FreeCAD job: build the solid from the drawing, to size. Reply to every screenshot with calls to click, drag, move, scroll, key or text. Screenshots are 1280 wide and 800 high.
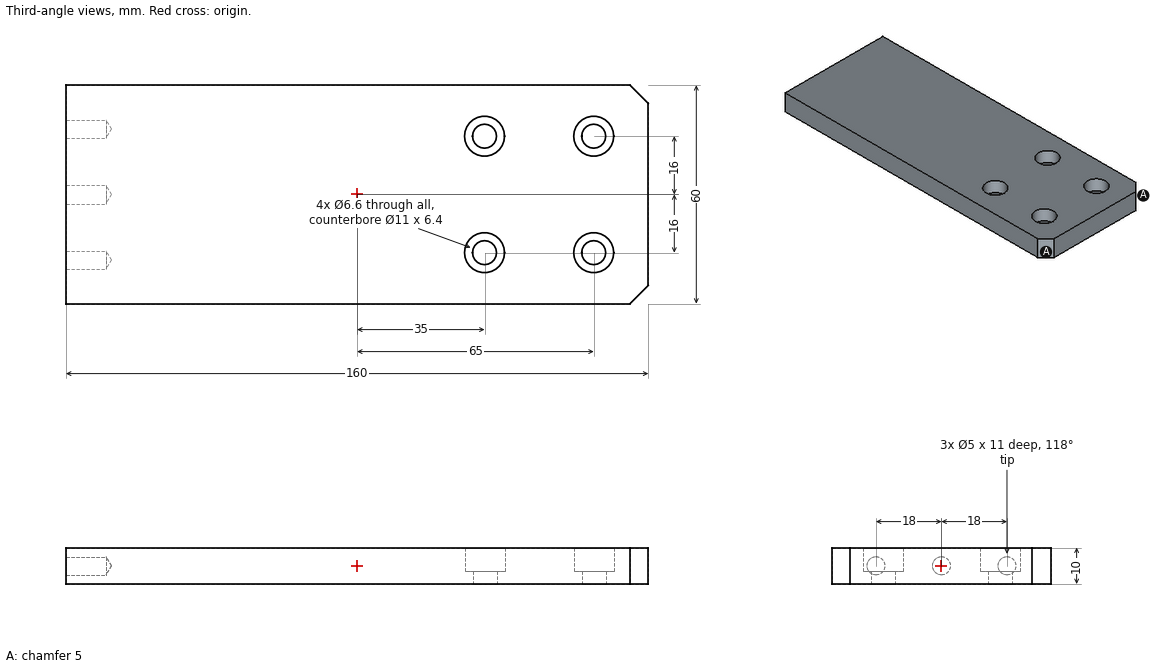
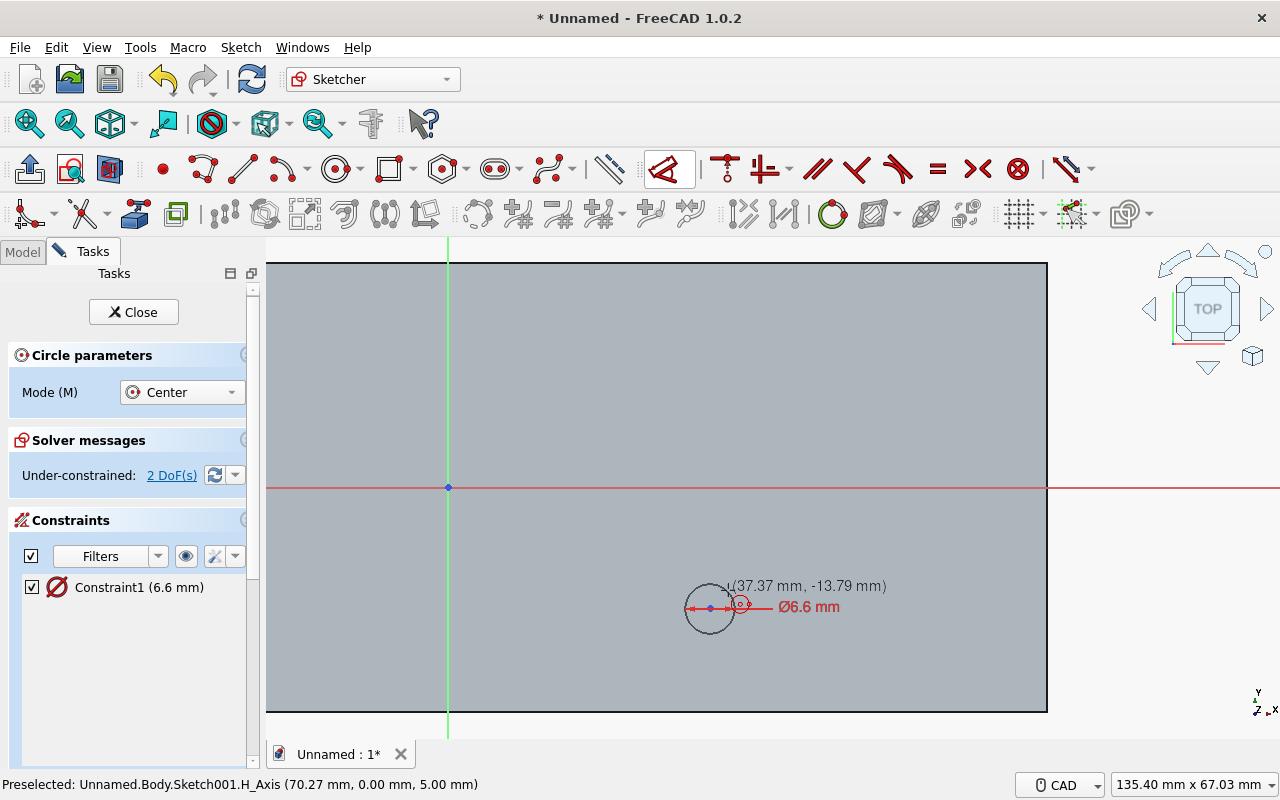
click(935, 608)
move(952, 590)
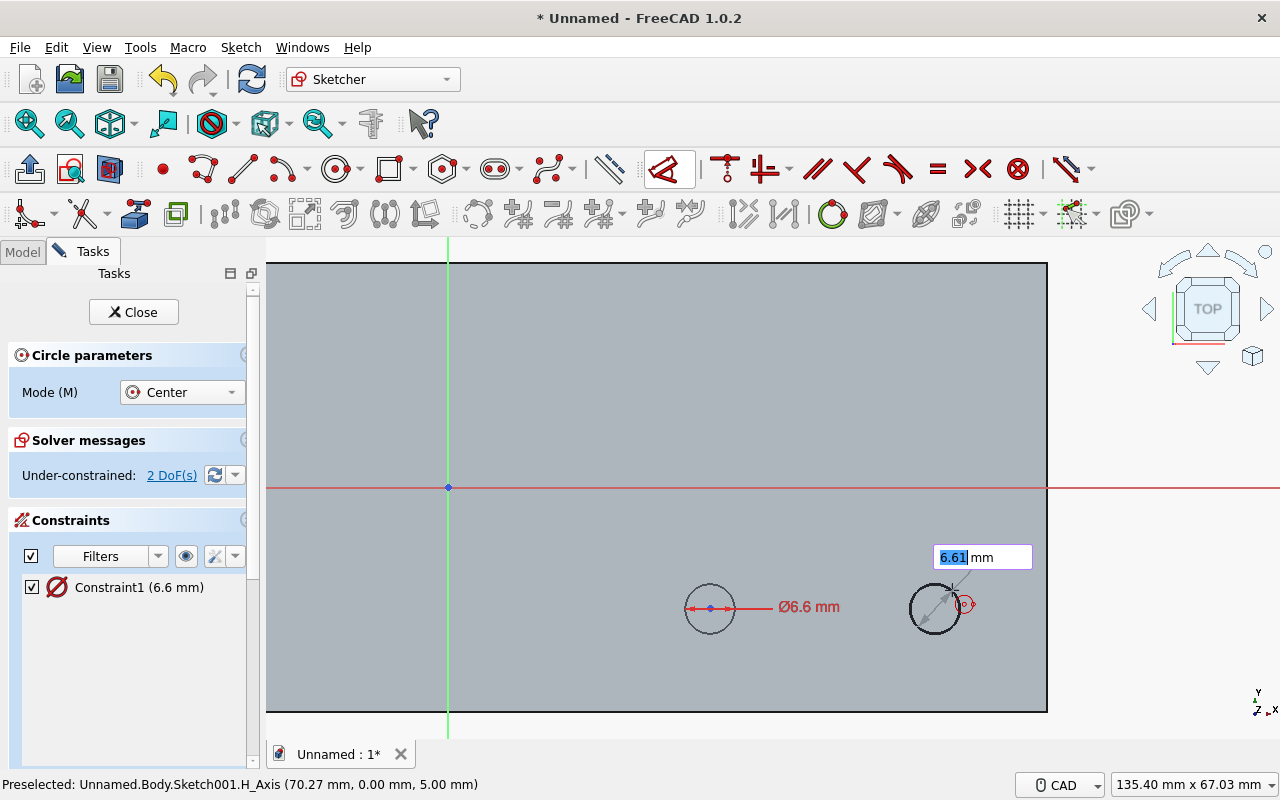
text(6.6)
key(Return)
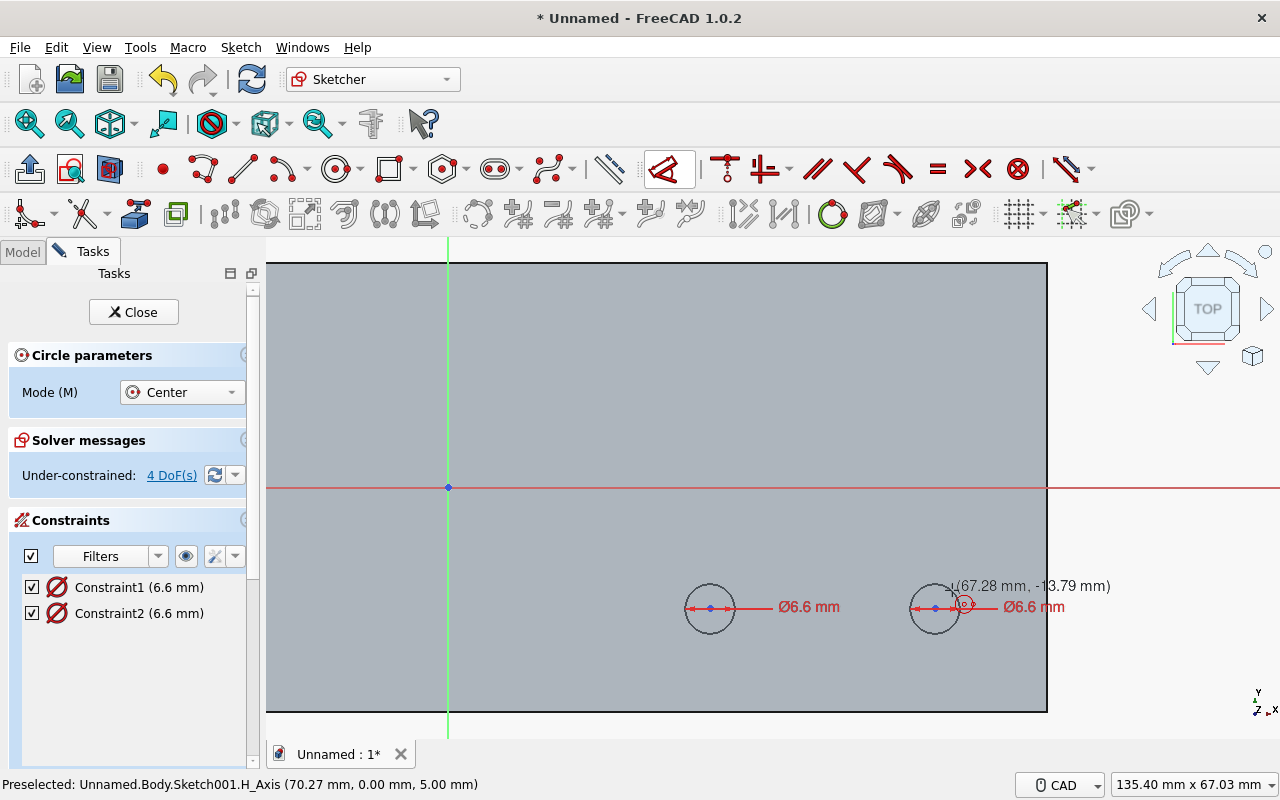
click(935, 368)
move(952, 350)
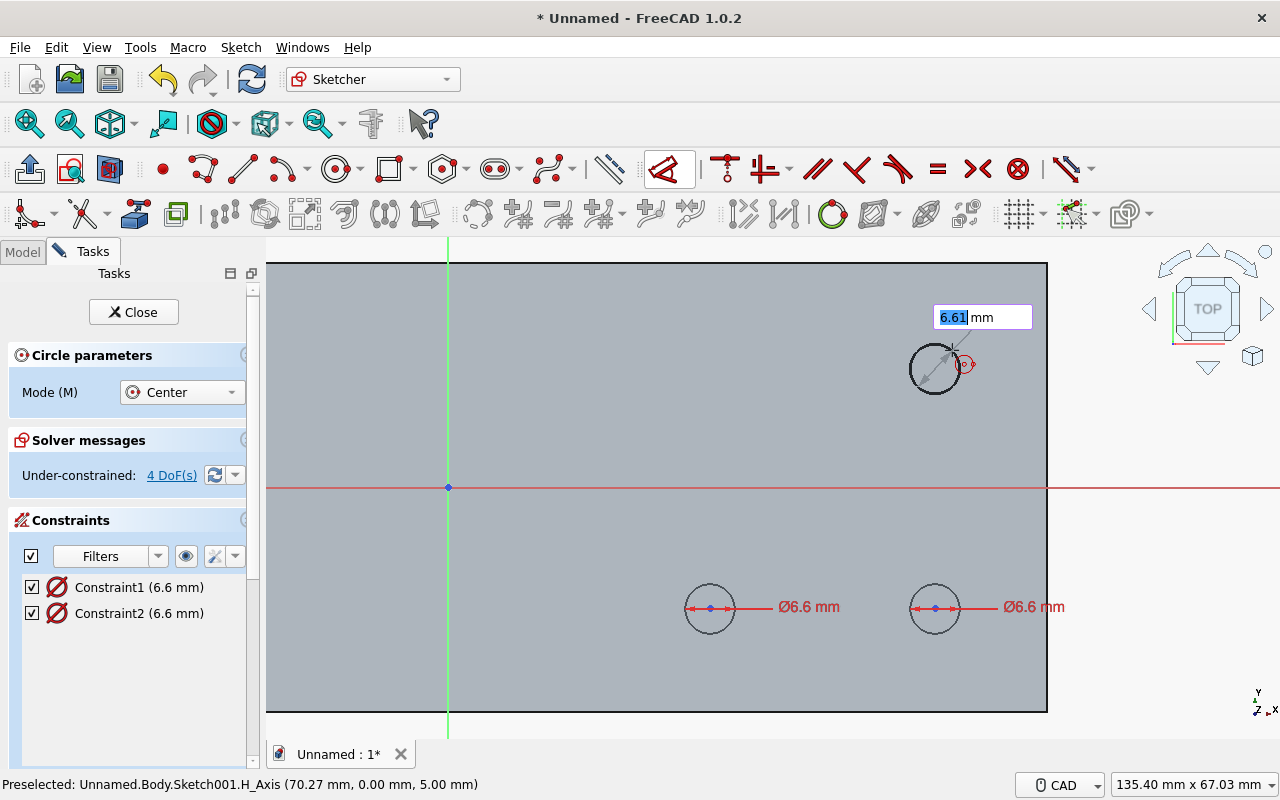
text(6.6)
key(Return)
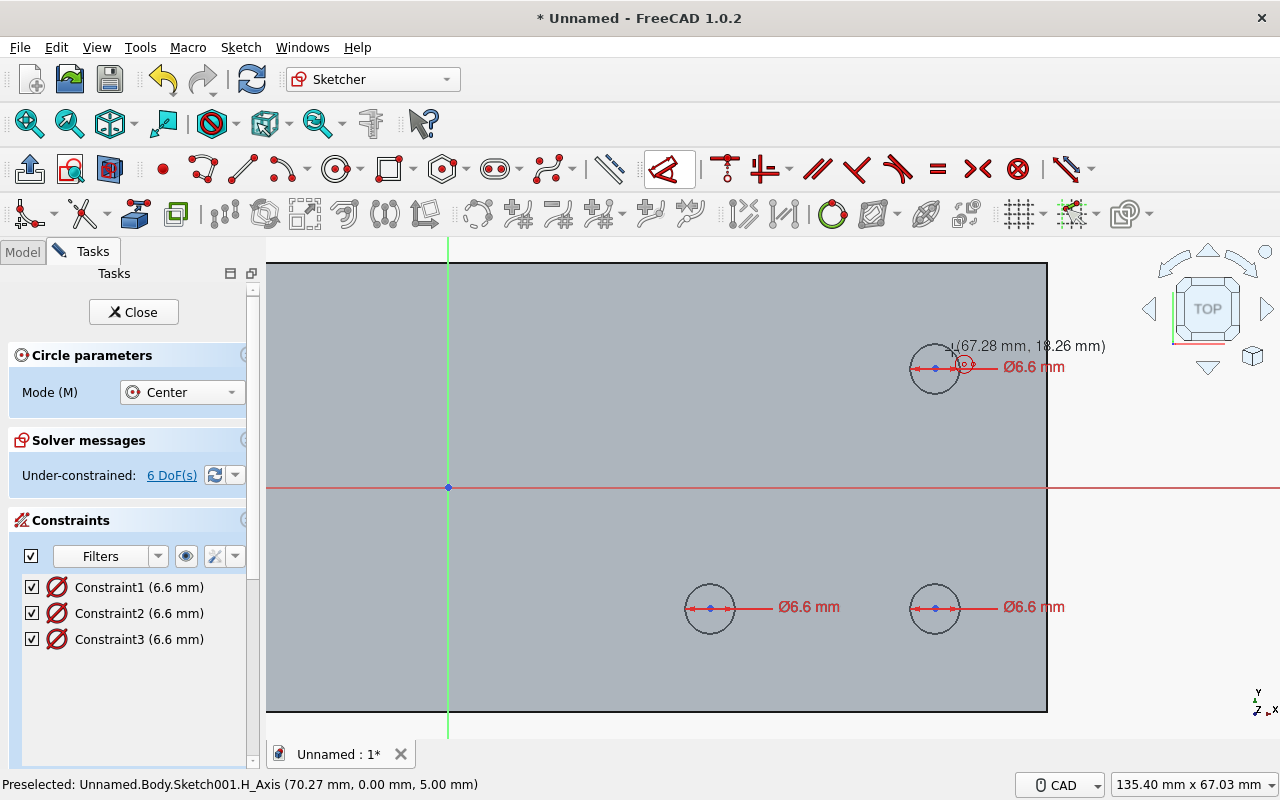
click(710, 368)
move(728, 350)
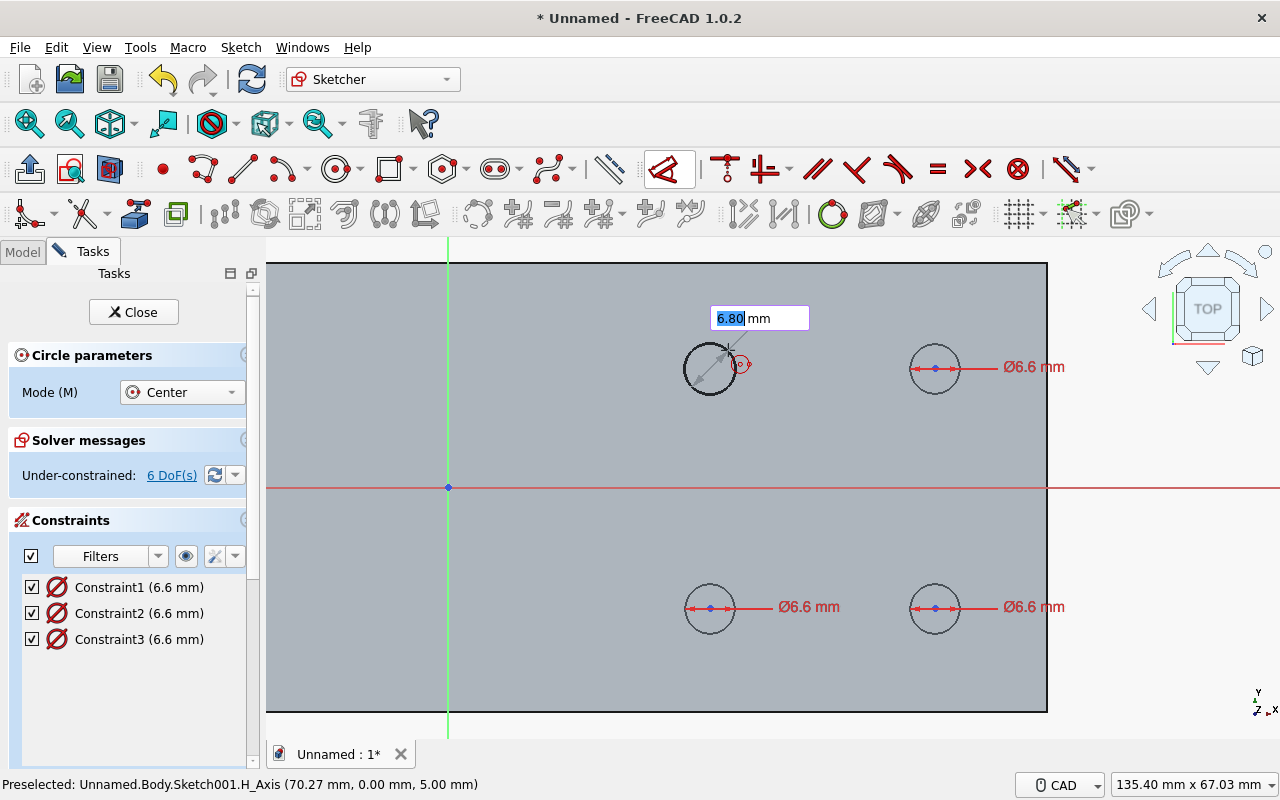
text(6.6)
key(Return)
key(Escape)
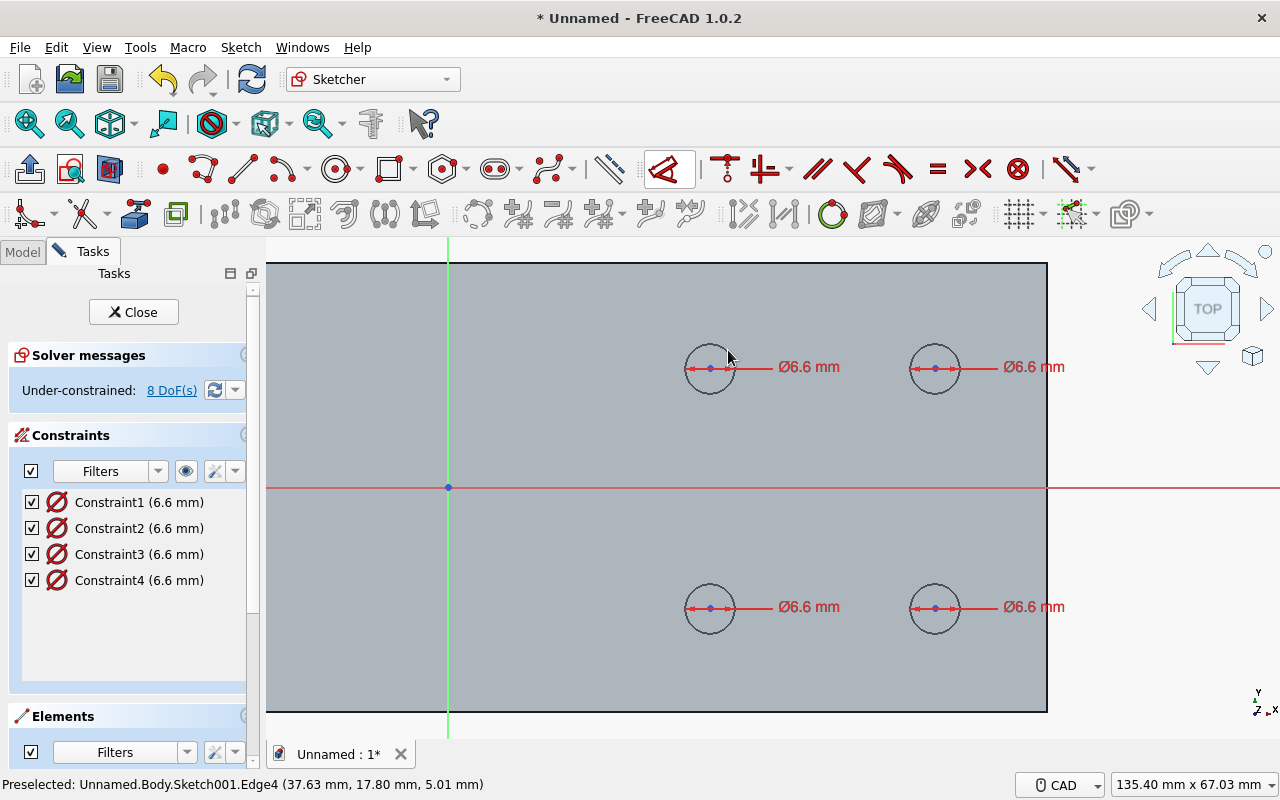
click(710, 609)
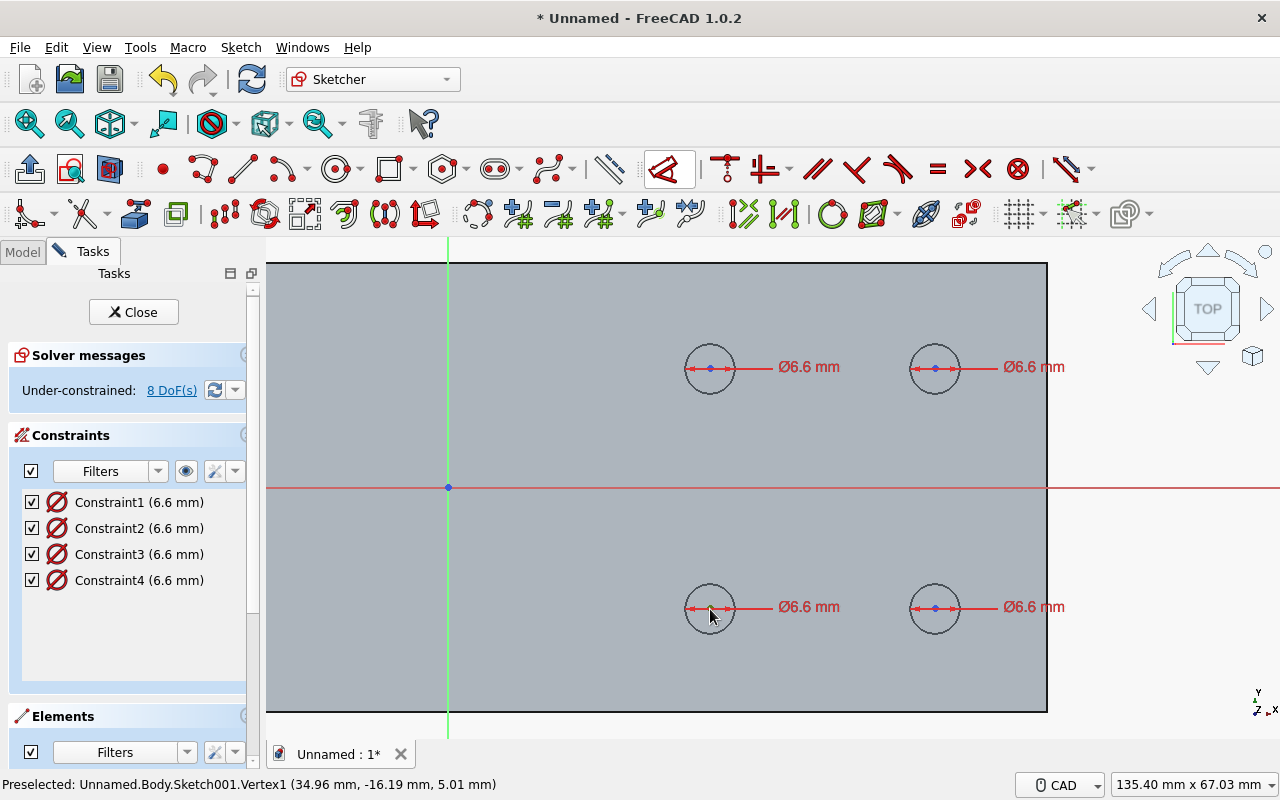
click(935, 609)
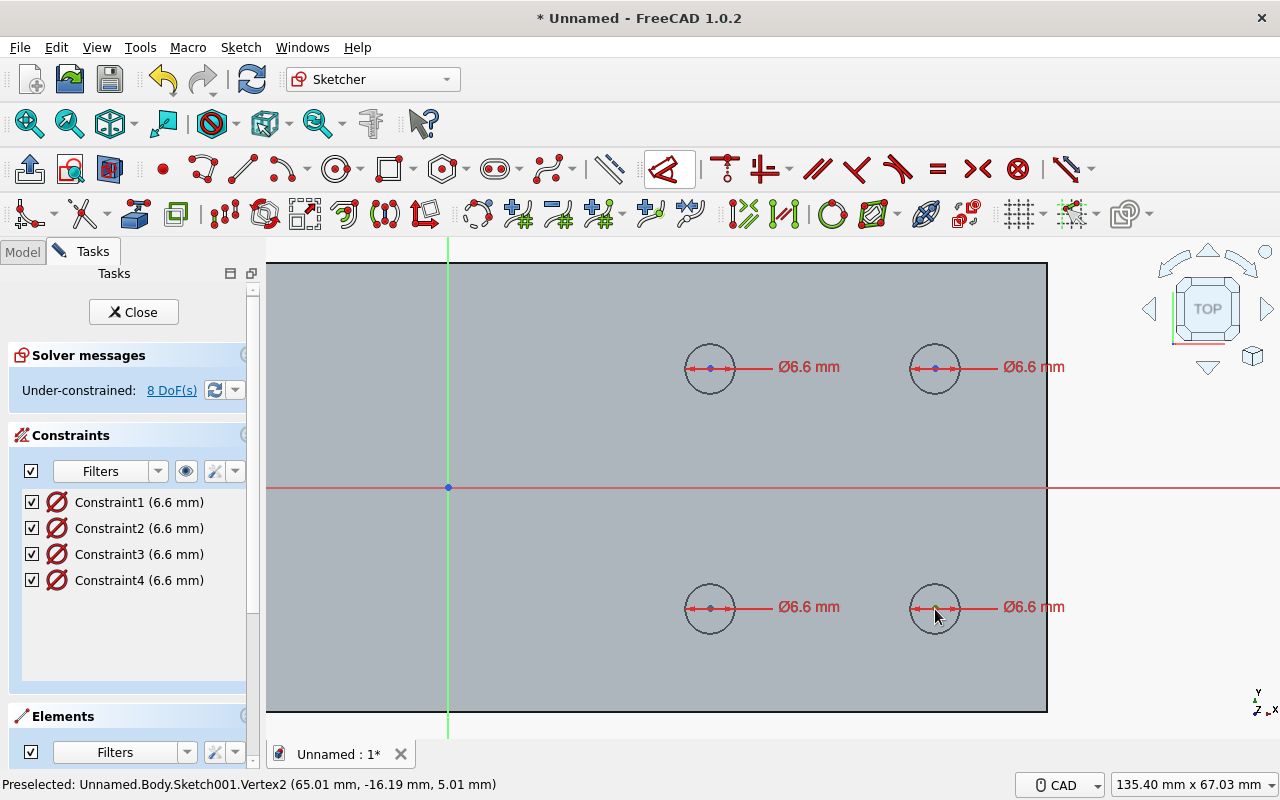
key(h)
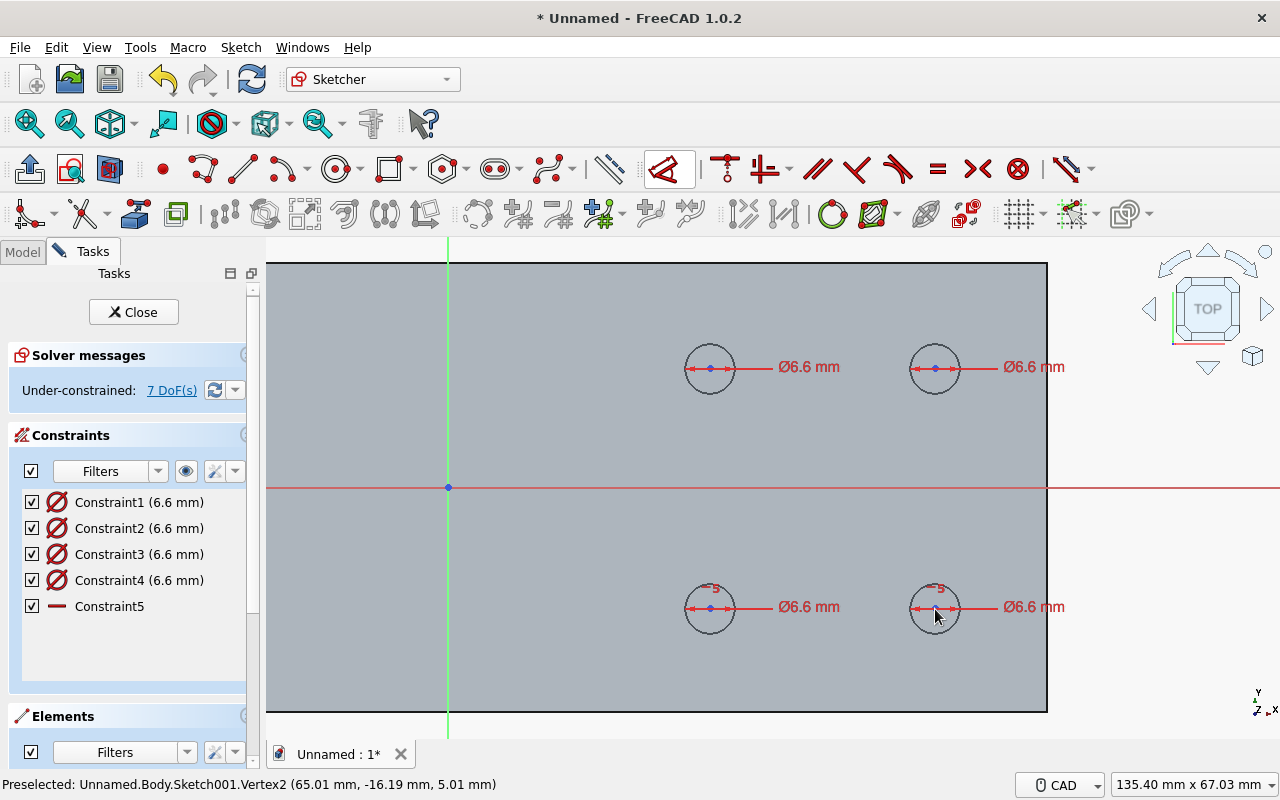
click(935, 609)